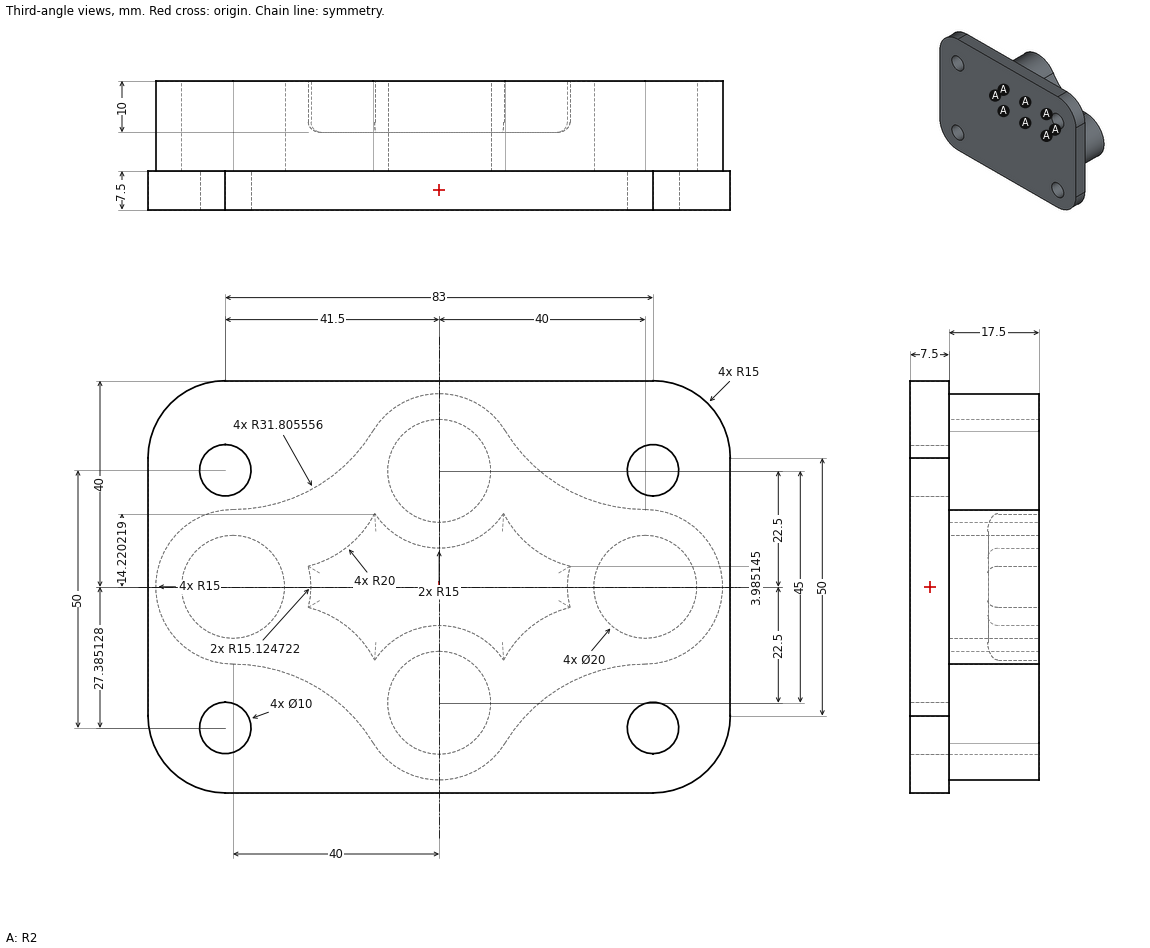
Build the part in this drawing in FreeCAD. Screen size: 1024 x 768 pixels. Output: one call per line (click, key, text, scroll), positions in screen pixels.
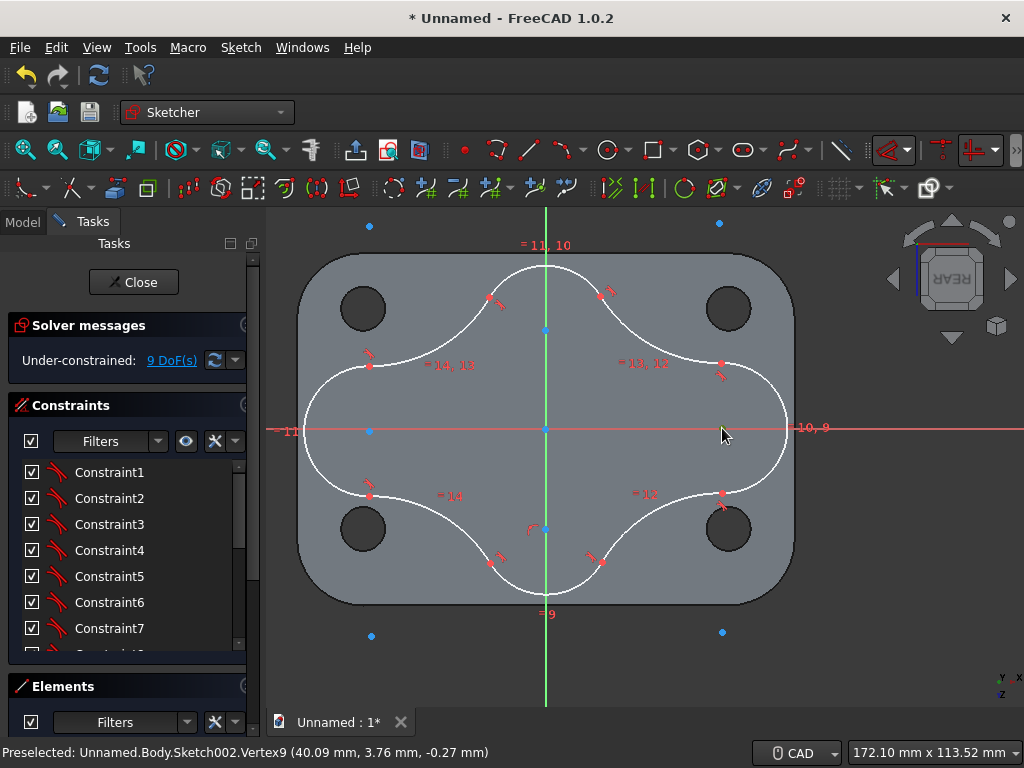
click(334, 429)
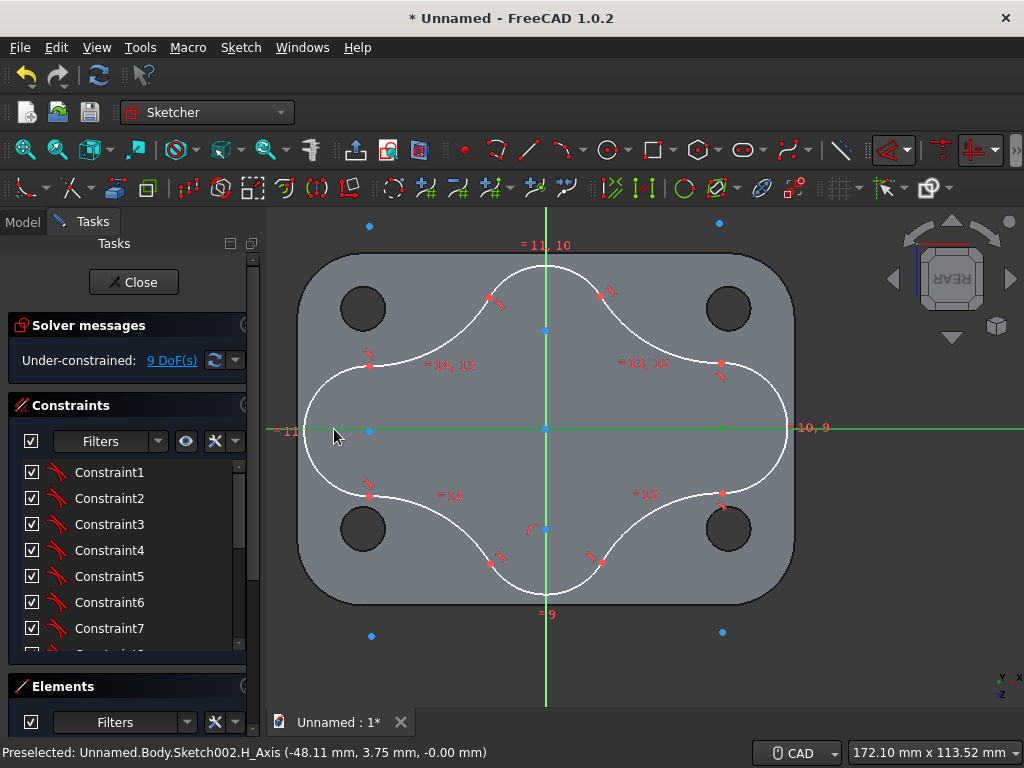
click(942, 150)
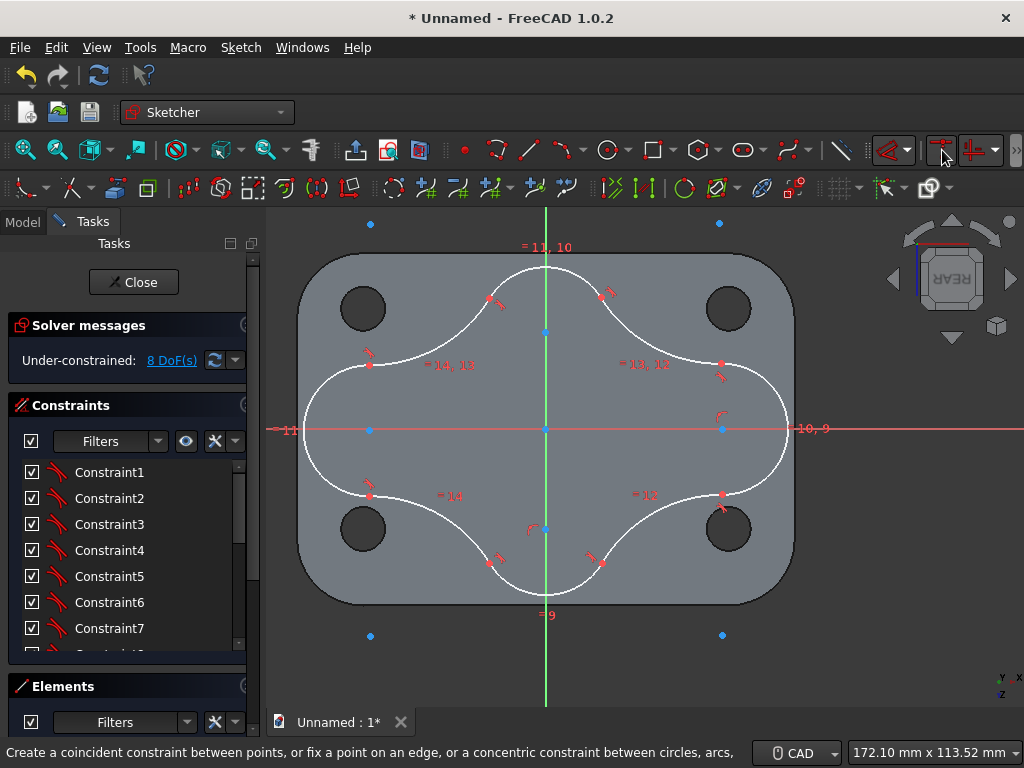
click(545, 333)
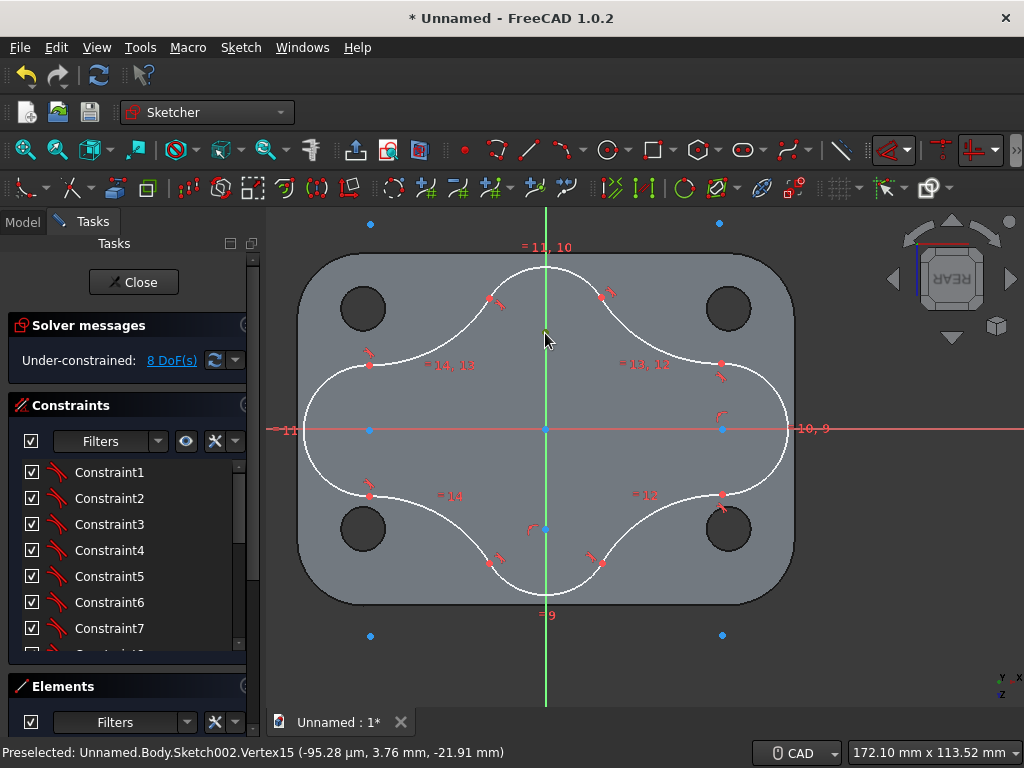
click(546, 647)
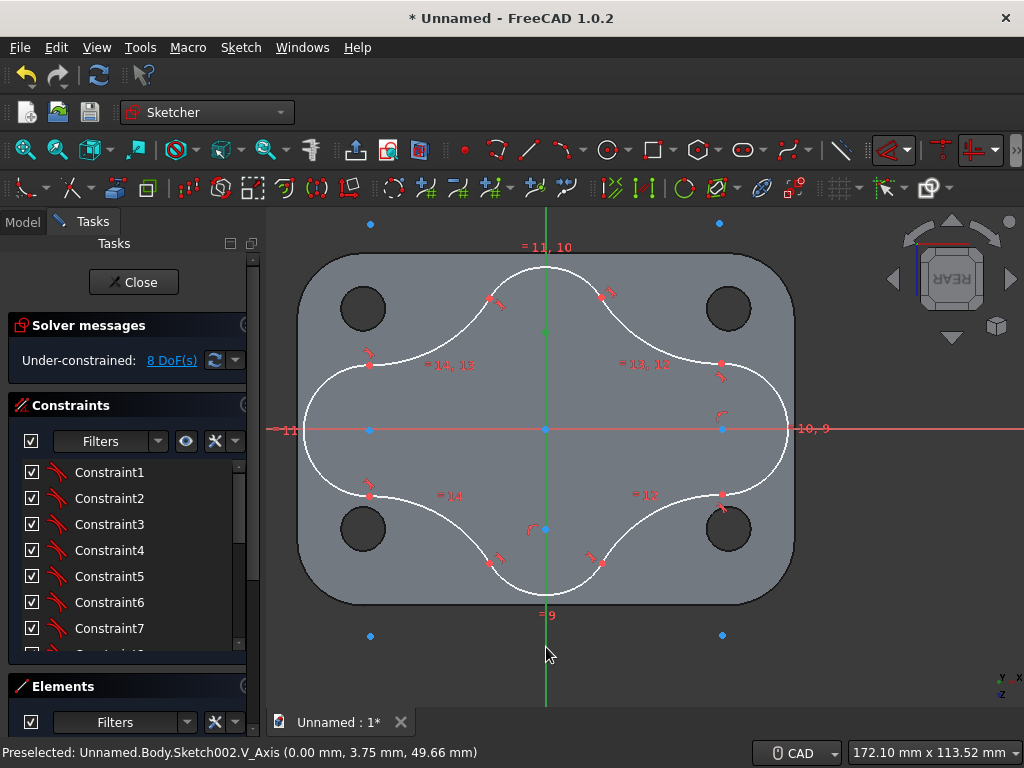
key(c)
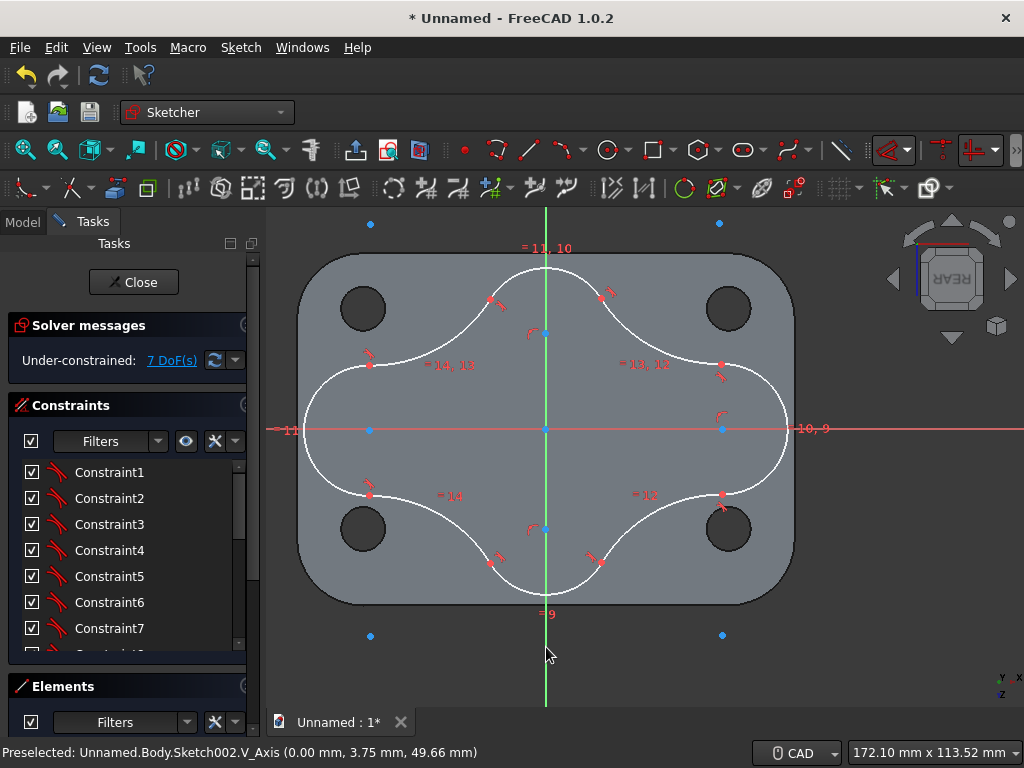
click(369, 431)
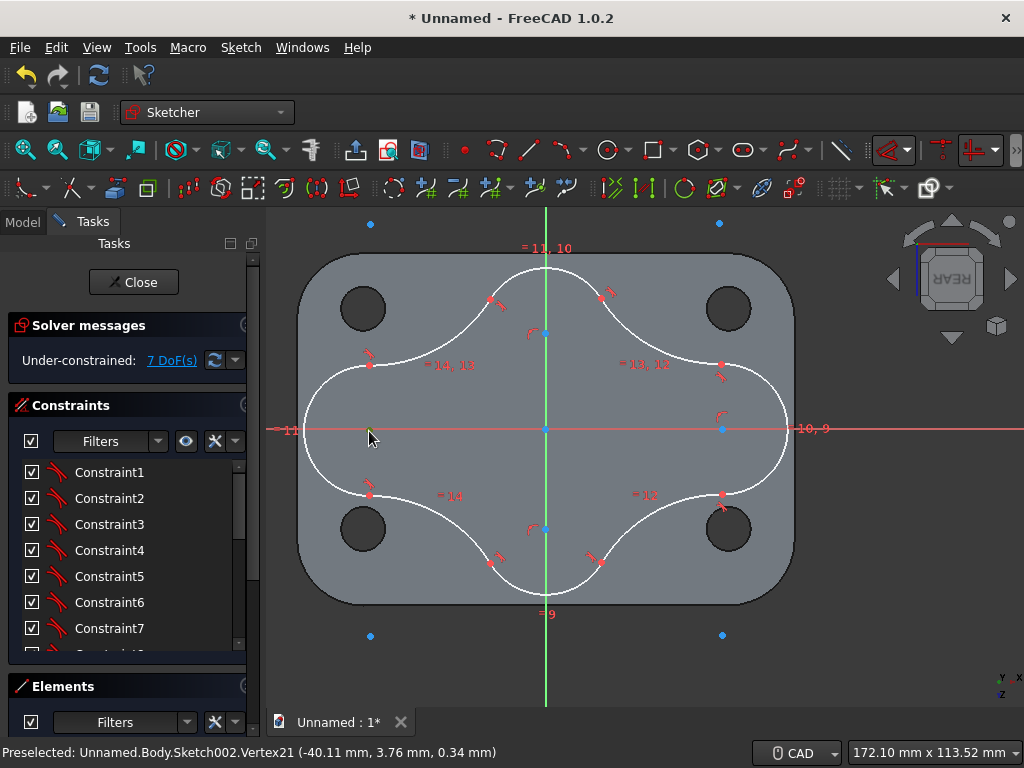
click(334, 429)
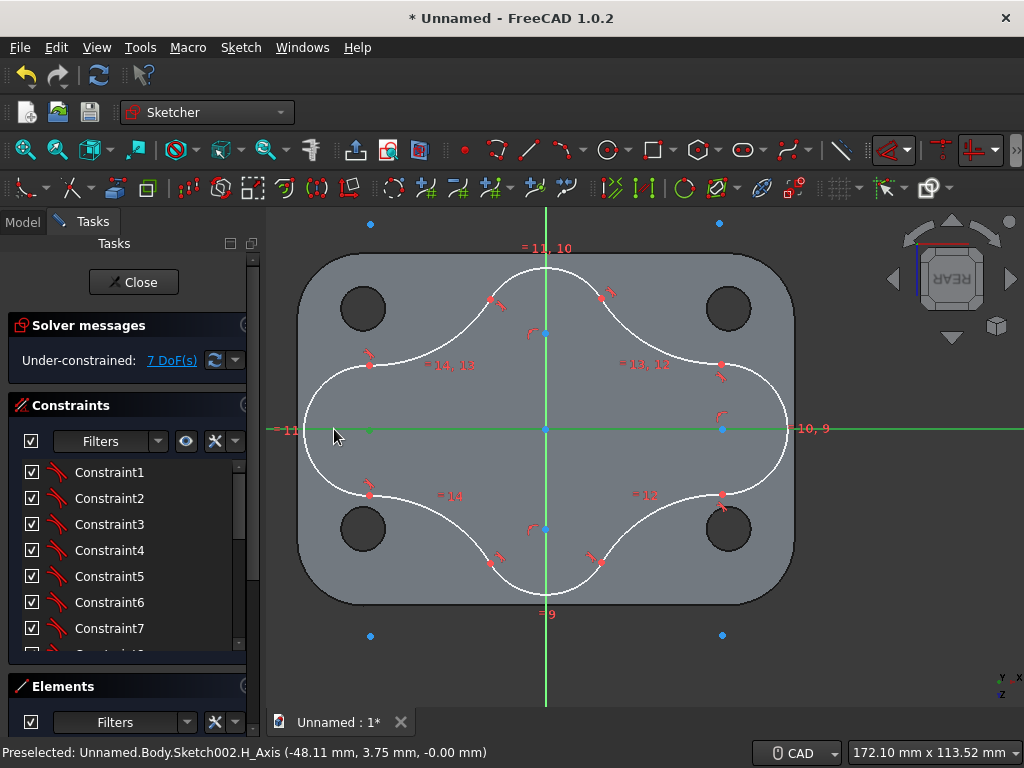
click(942, 150)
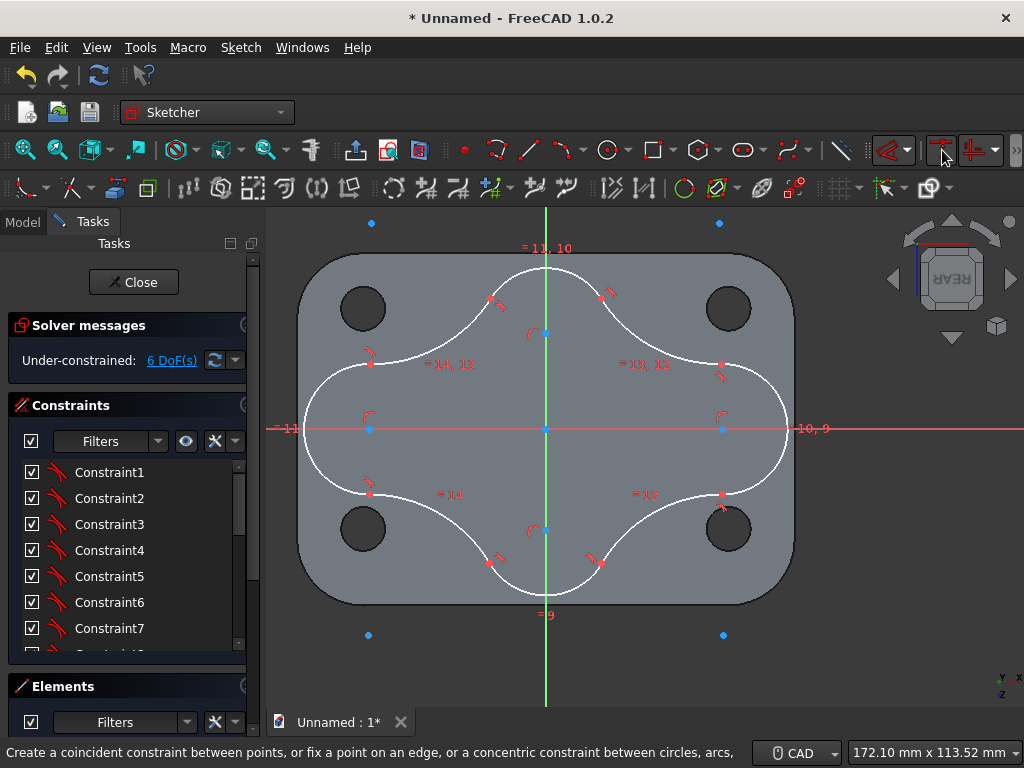
click(520, 590)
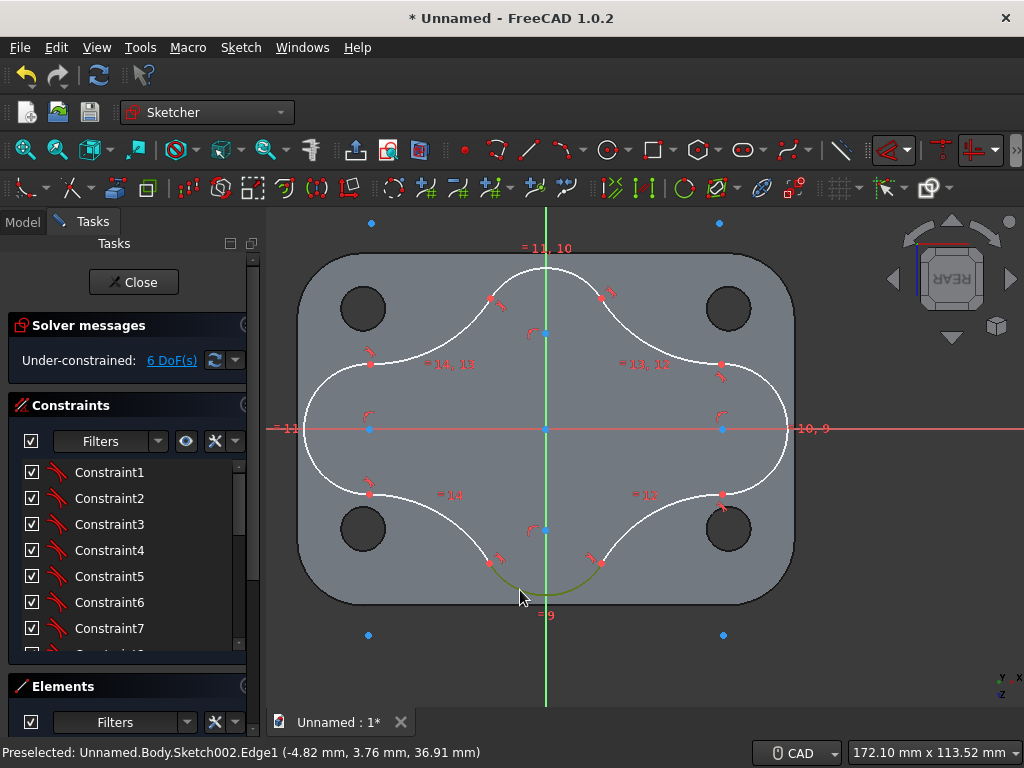
click(910, 150)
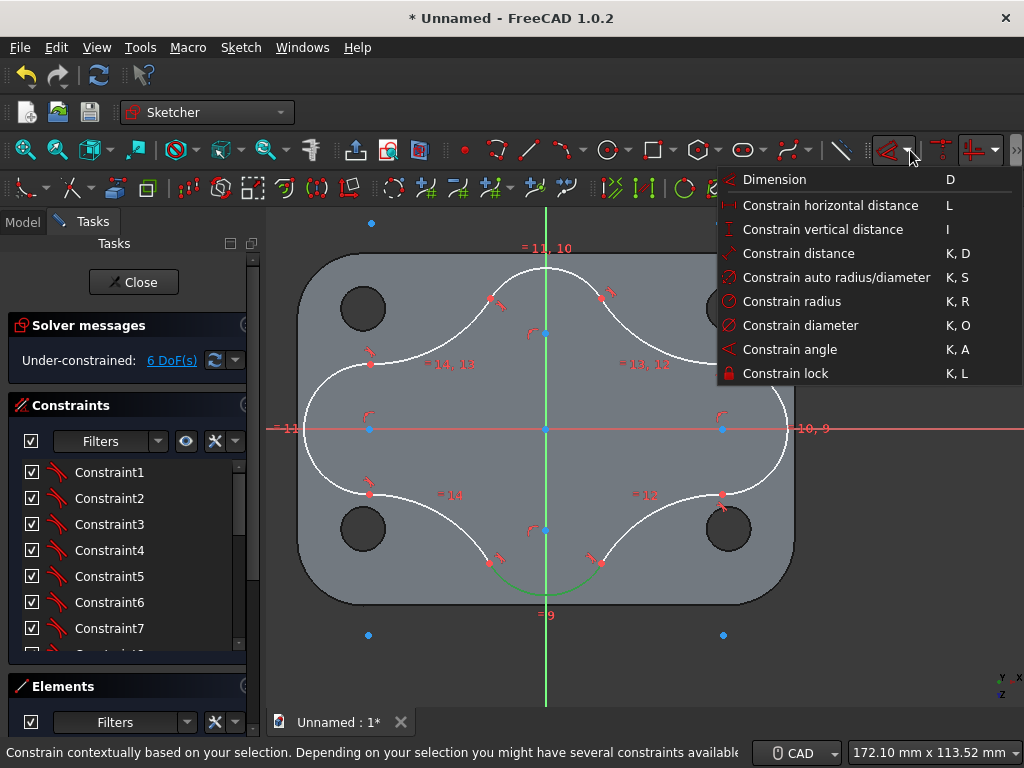
click(870, 301)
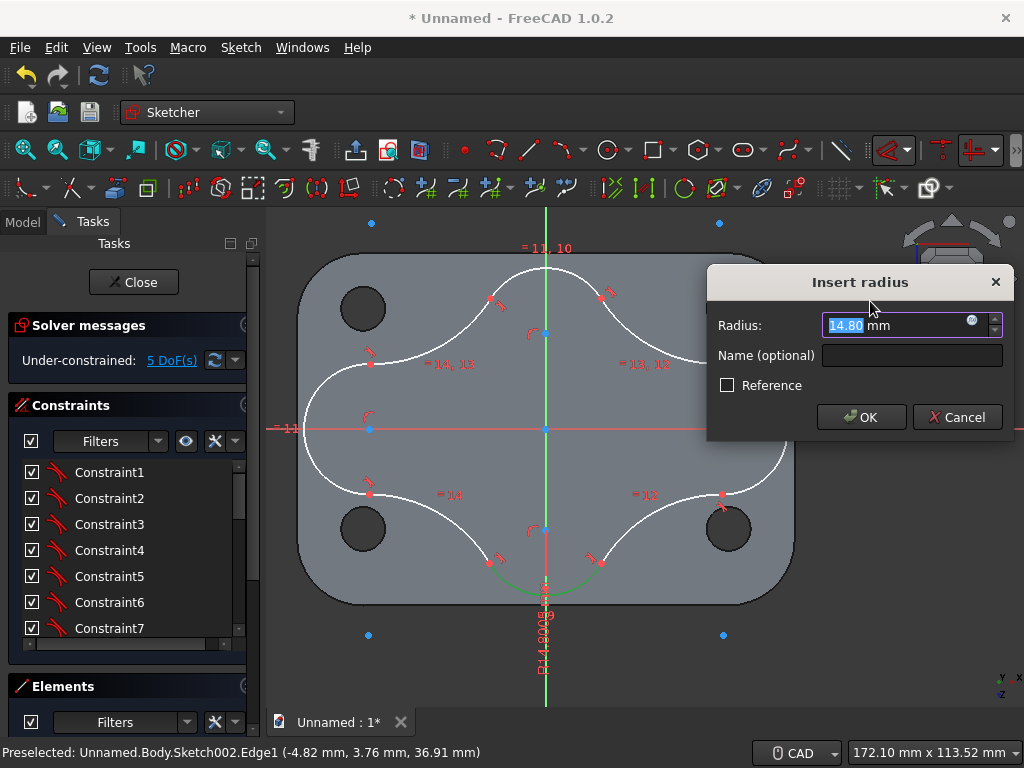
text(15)
key(Return)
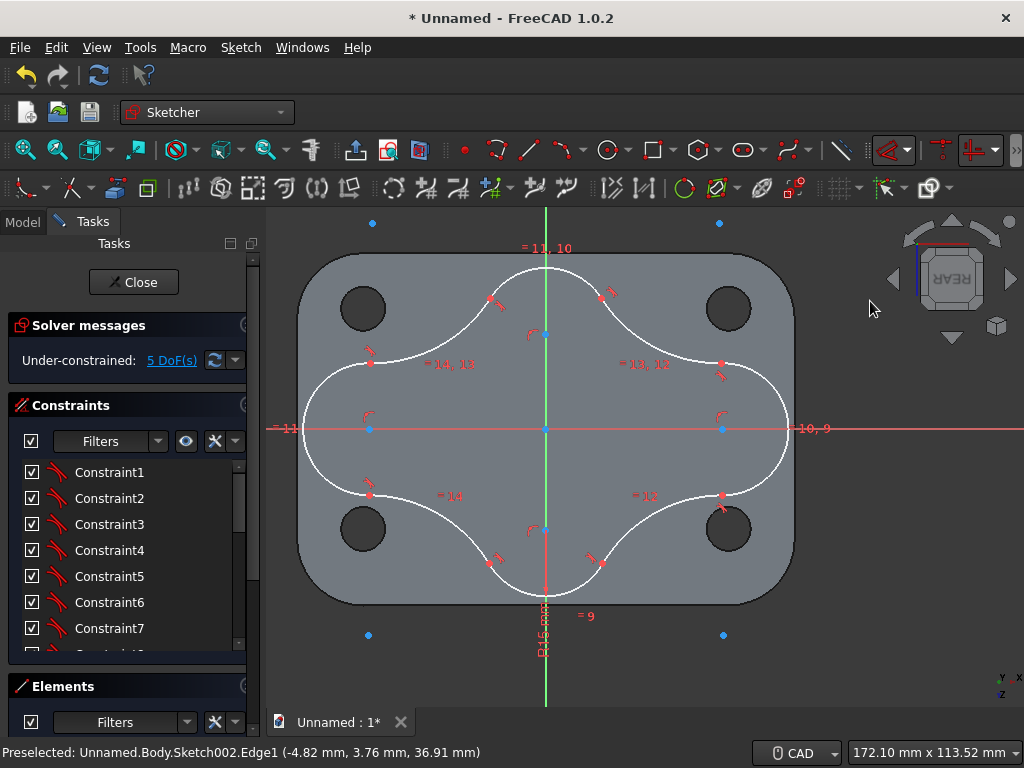
click(680, 502)